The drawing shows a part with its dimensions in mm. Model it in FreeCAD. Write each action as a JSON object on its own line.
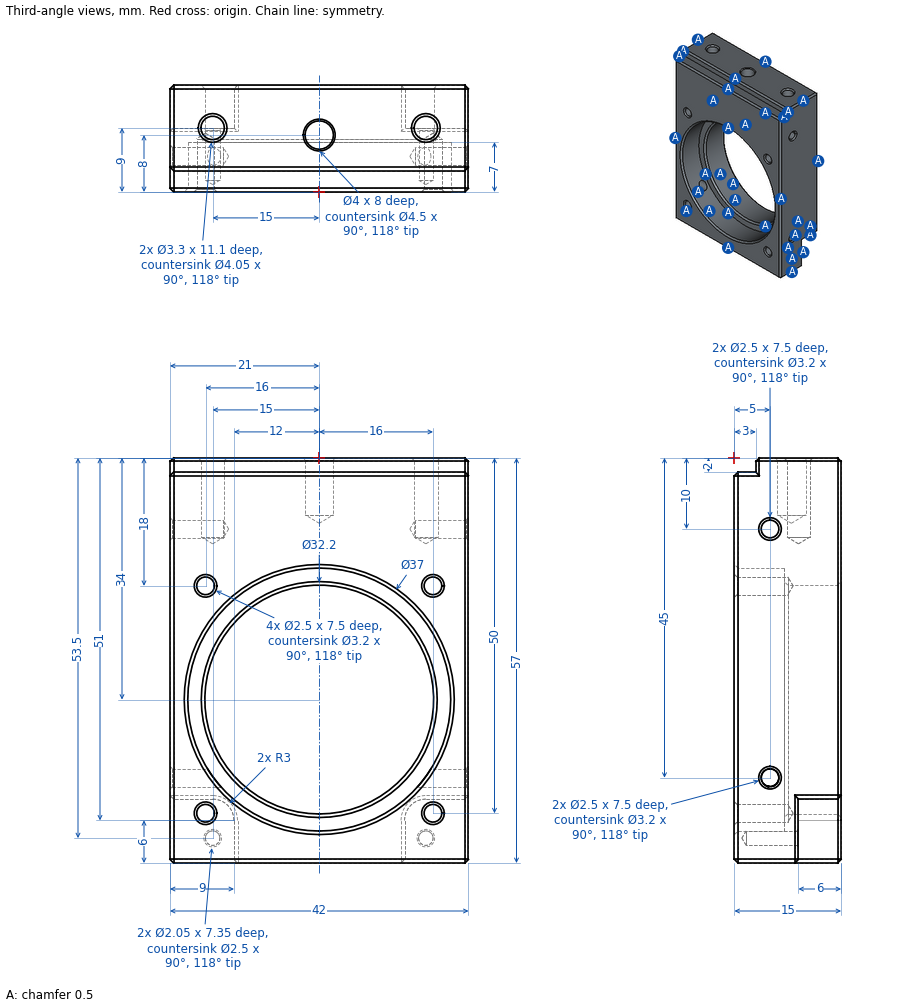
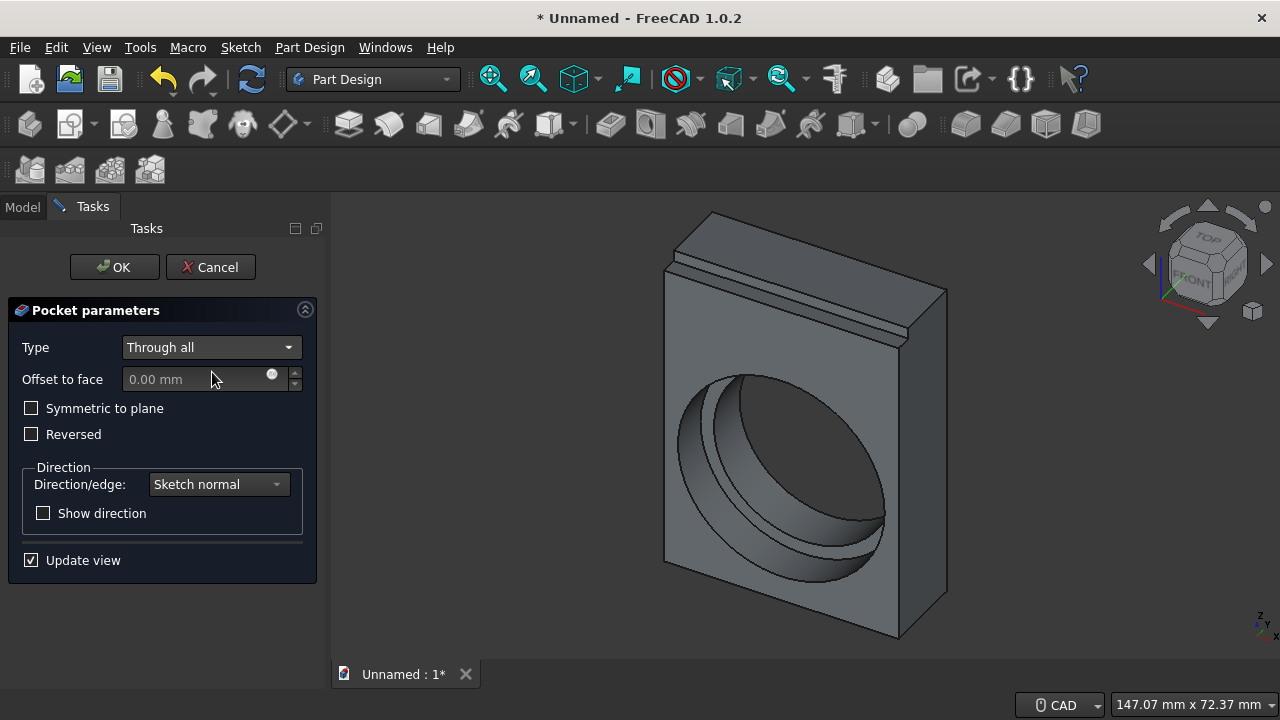
{"action": "left_click", "coordinate": [115, 267]}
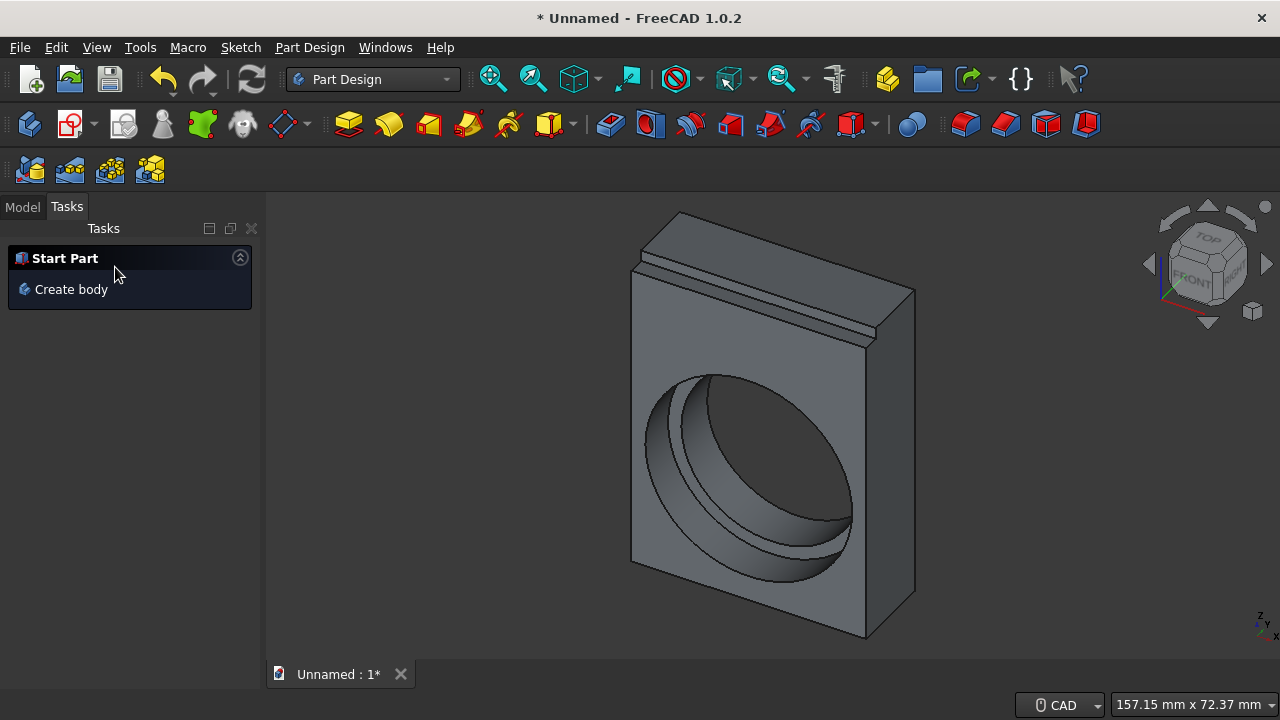
{"action": "left_click", "coordinate": [70, 124]}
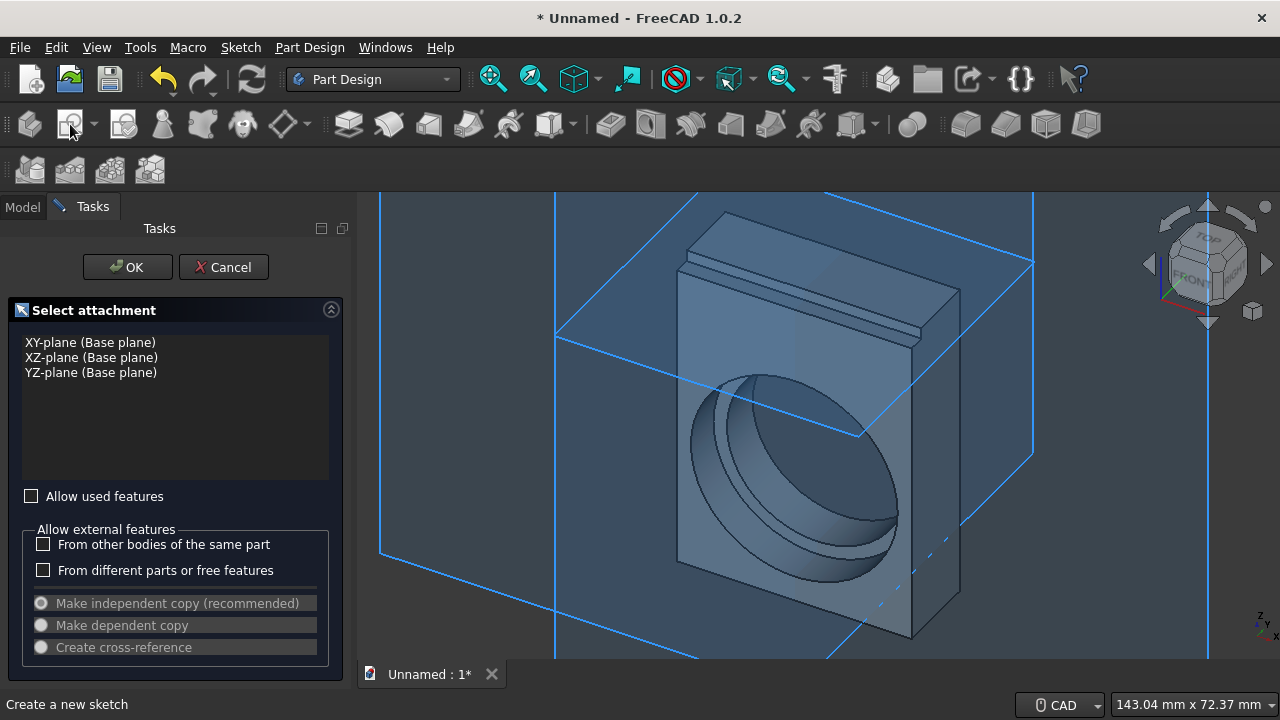
{"action": "left_click", "coordinate": [82, 342]}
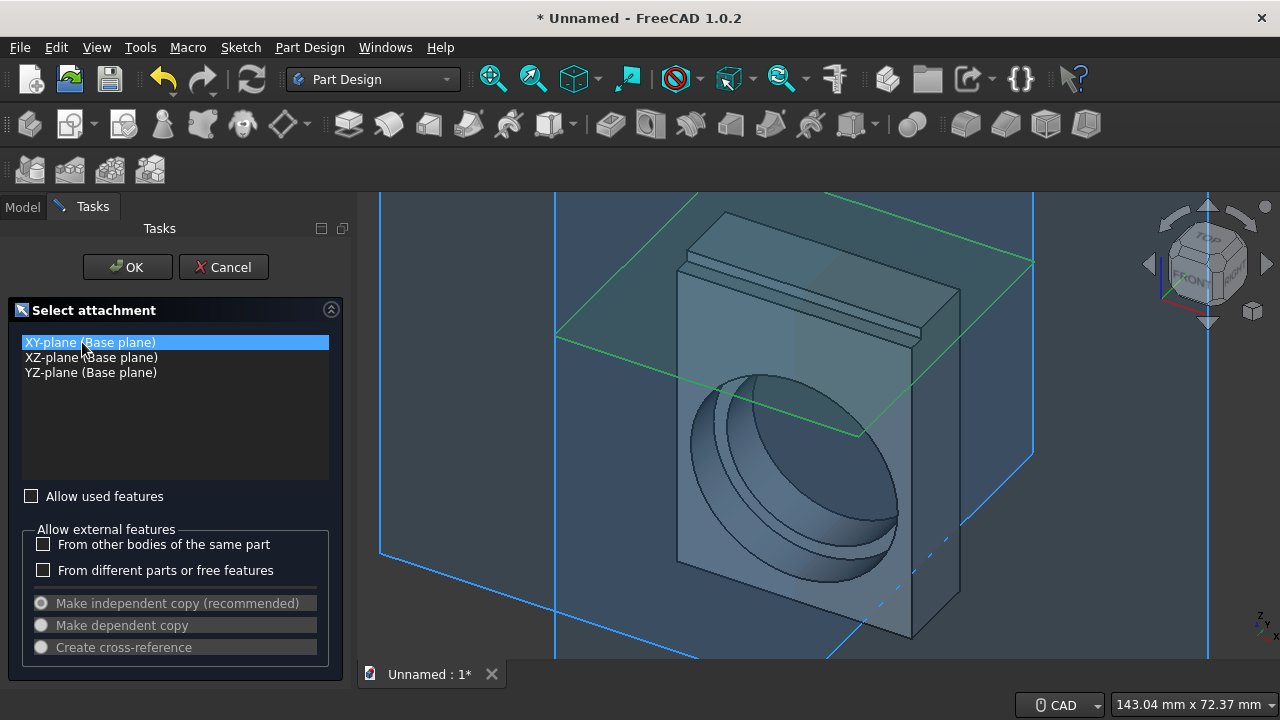
{"action": "left_click", "coordinate": [128, 267]}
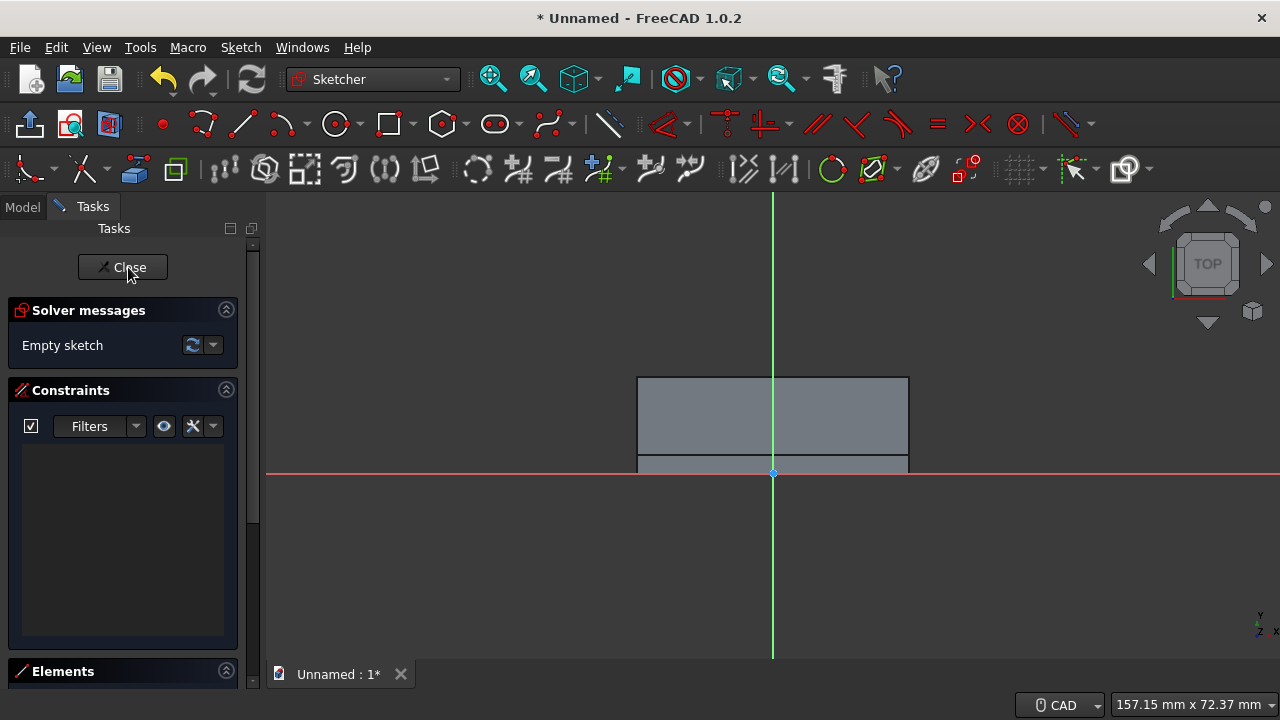
{"action": "scroll", "coordinate": [813, 448], "scroll_direction": "up", "scroll_amount": 5}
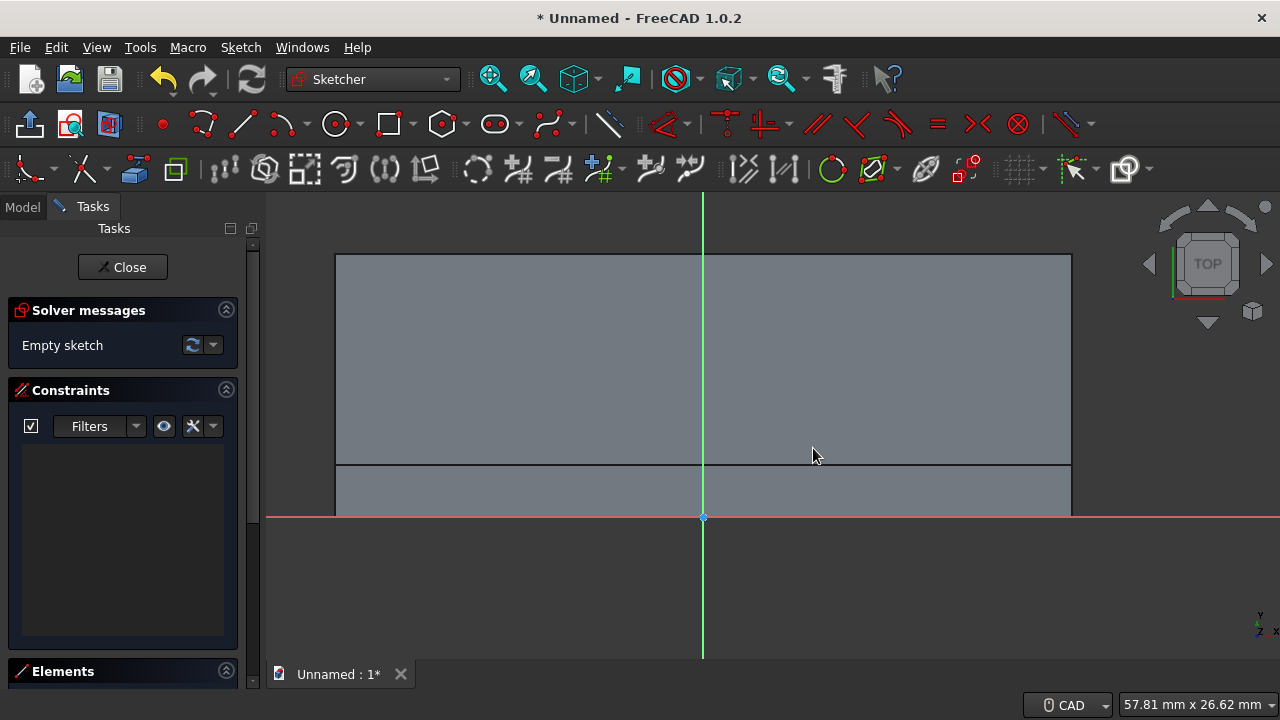
{"action": "left_click", "coordinate": [336, 124]}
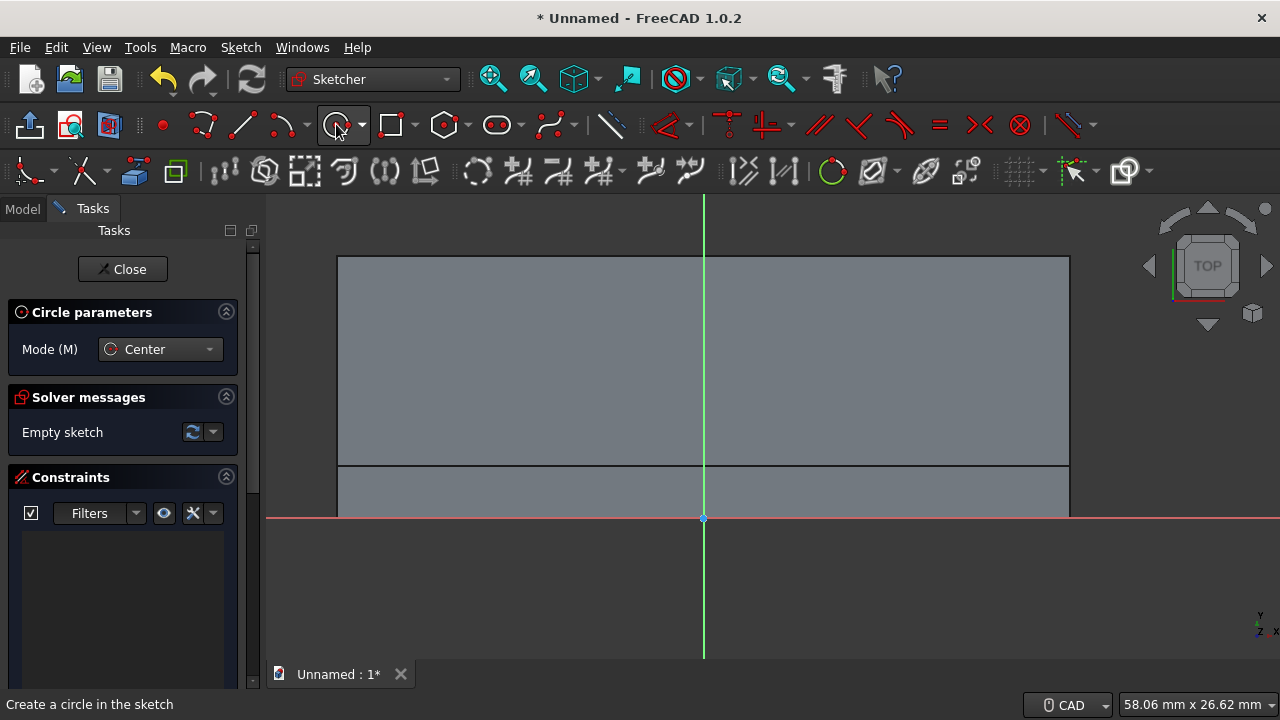
{"action": "left_click", "coordinate": [442, 361]}
{"action": "mouse_move", "coordinate": [462, 340]}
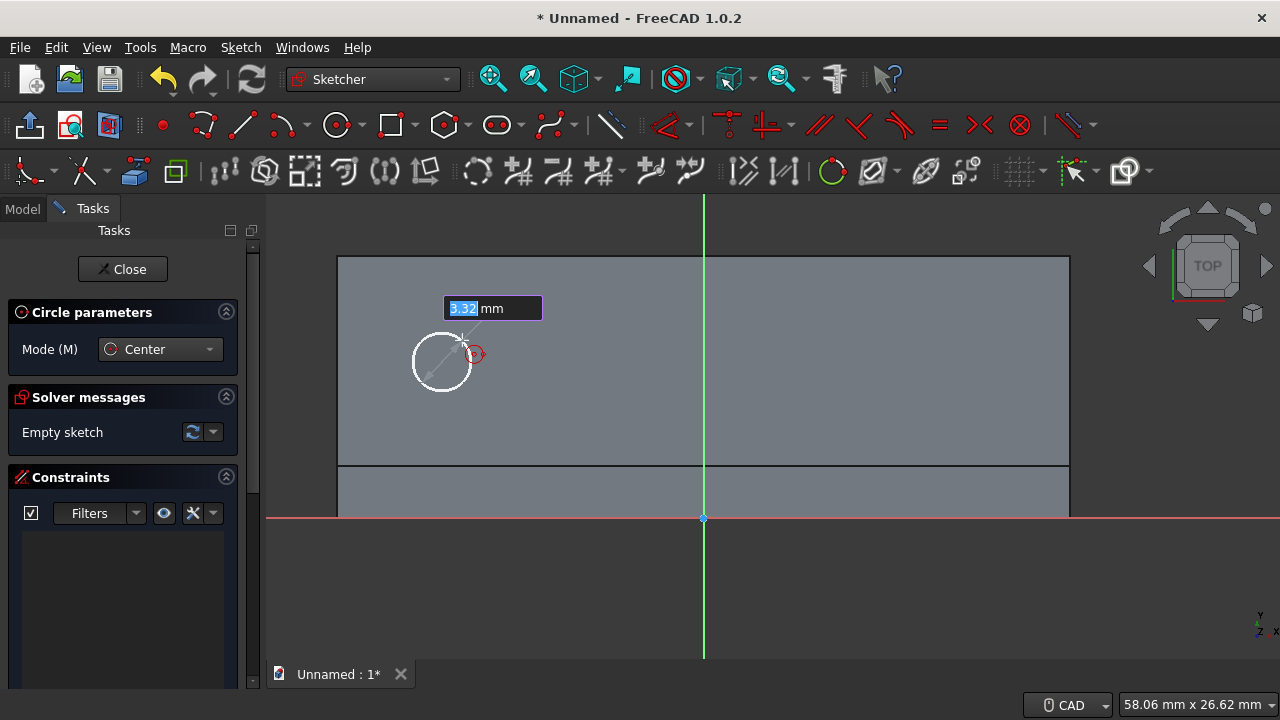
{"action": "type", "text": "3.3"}
{"action": "key", "text": "Return"}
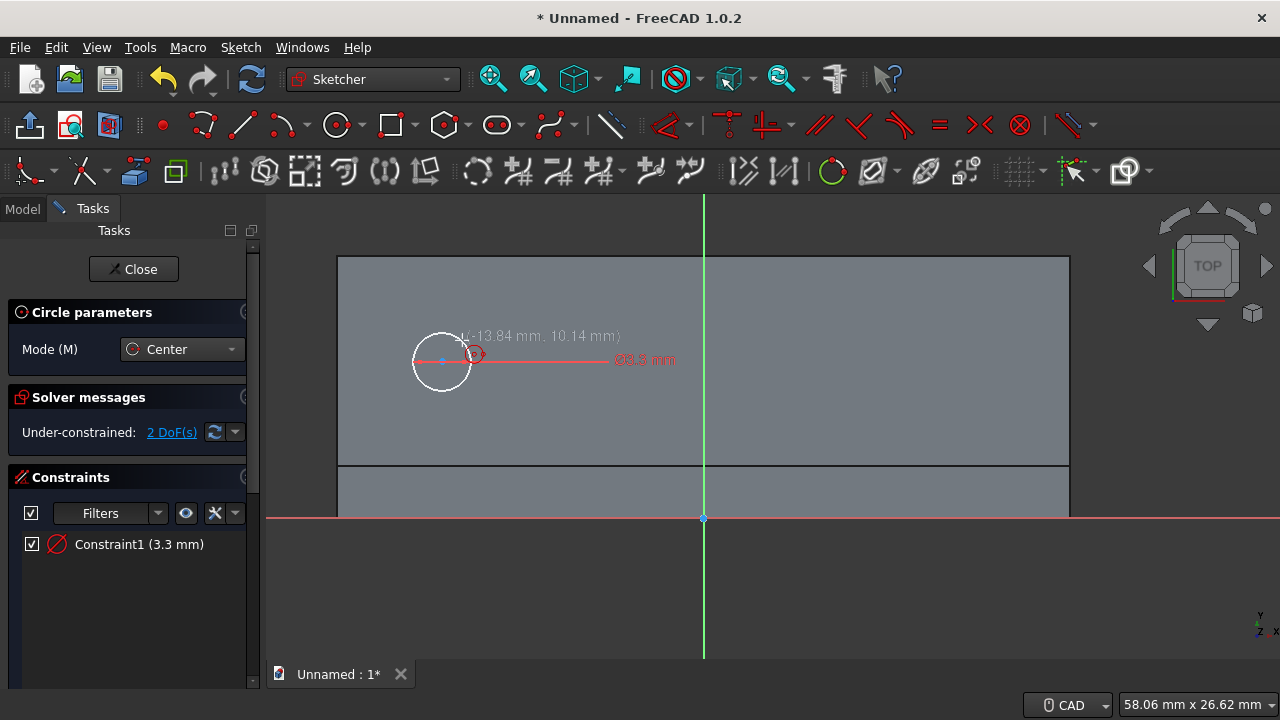
{"action": "left_click", "coordinate": [966, 361]}
{"action": "mouse_move", "coordinate": [986, 340]}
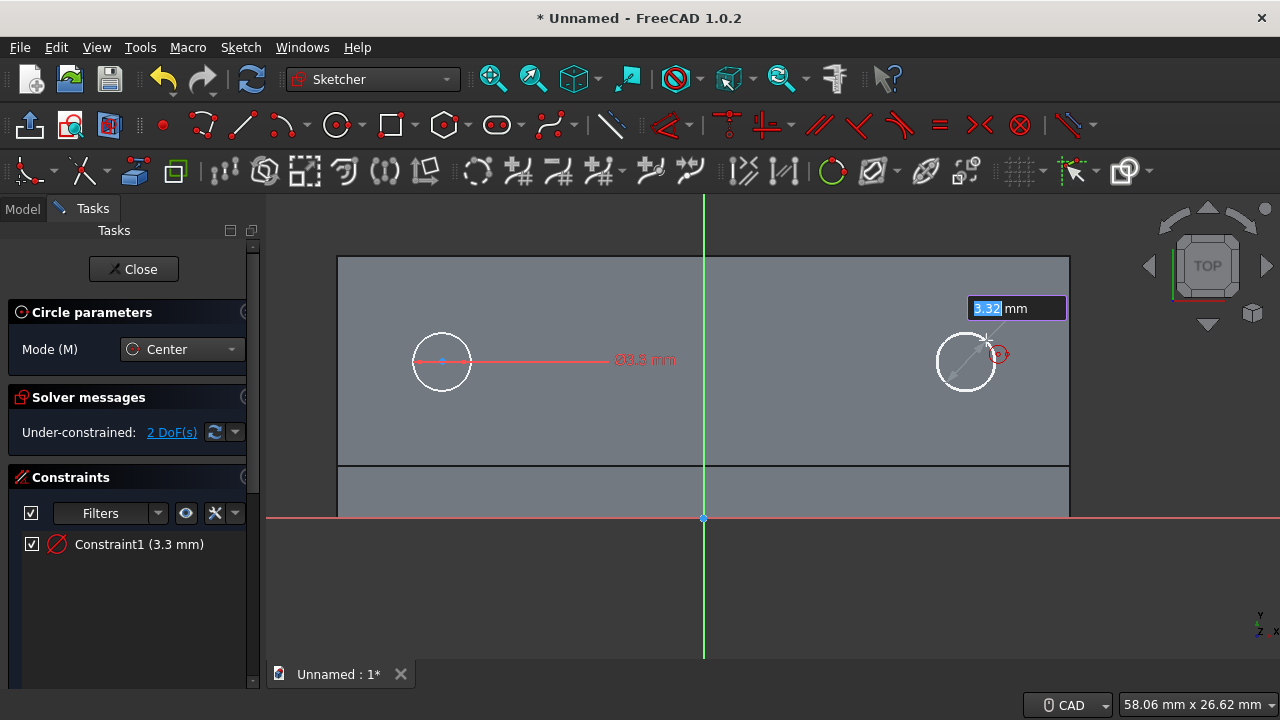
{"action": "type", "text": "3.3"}
{"action": "key", "text": "Return"}
{"action": "key", "text": "Escape"}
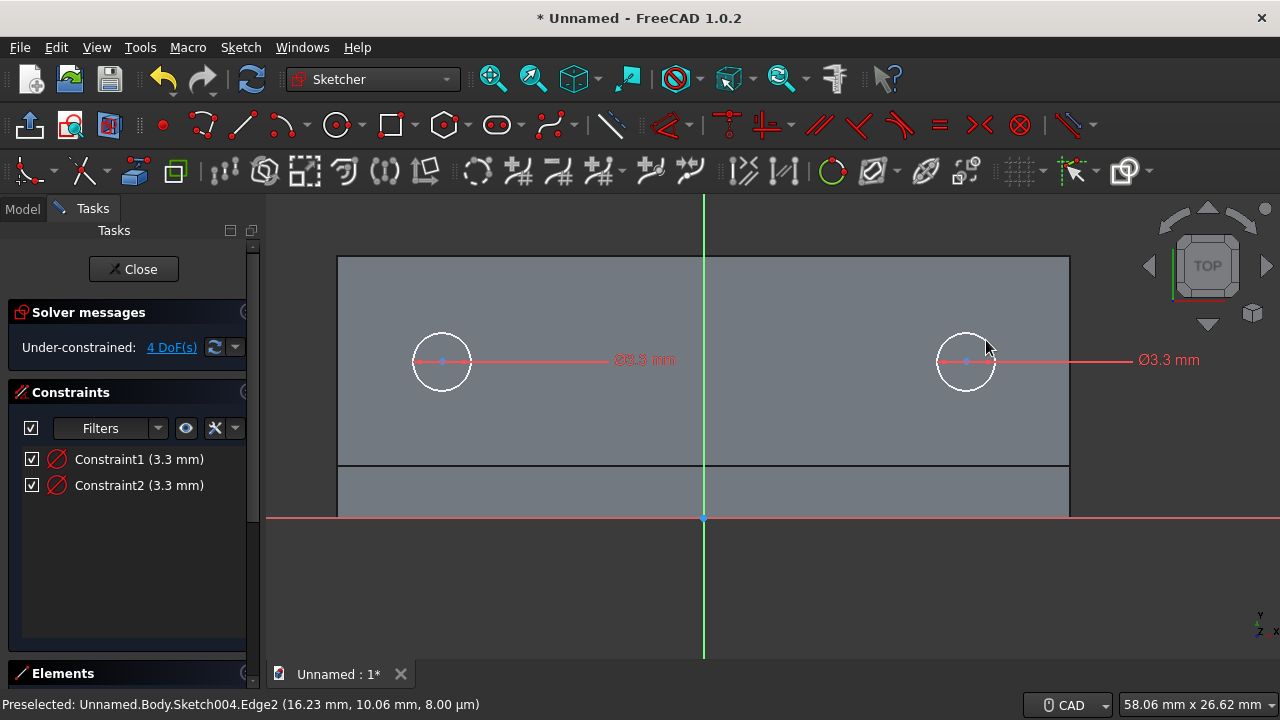
{"action": "left_click", "coordinate": [442, 362]}